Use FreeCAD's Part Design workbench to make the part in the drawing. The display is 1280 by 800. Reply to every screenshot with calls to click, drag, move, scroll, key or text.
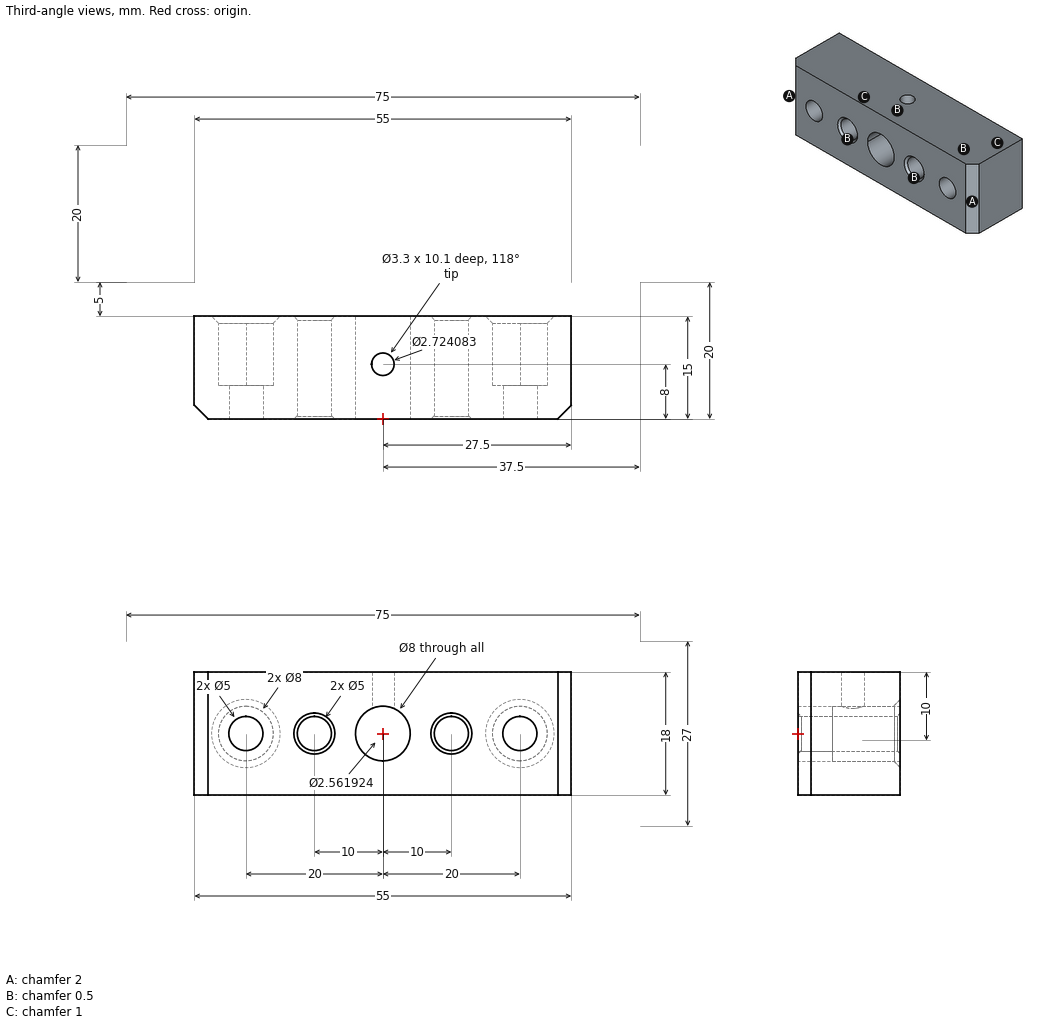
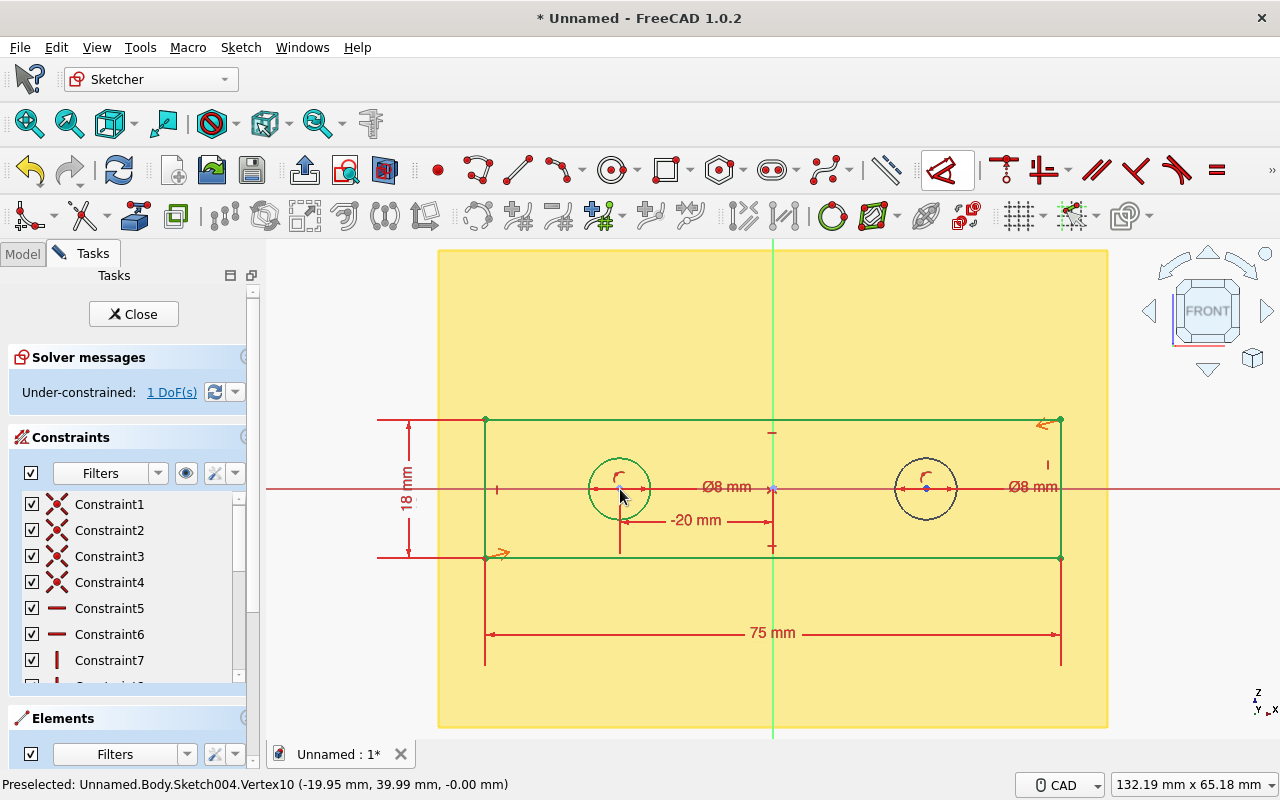
click(926, 489)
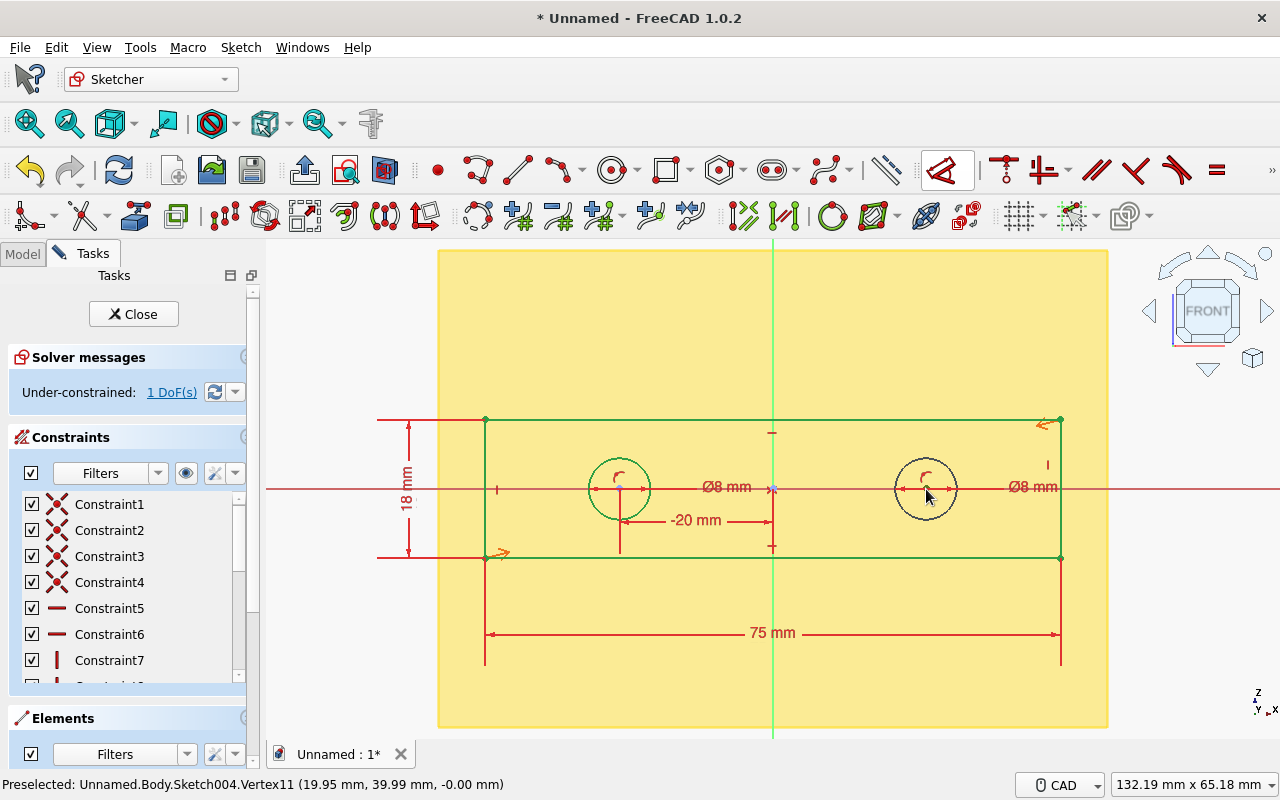
click(968, 170)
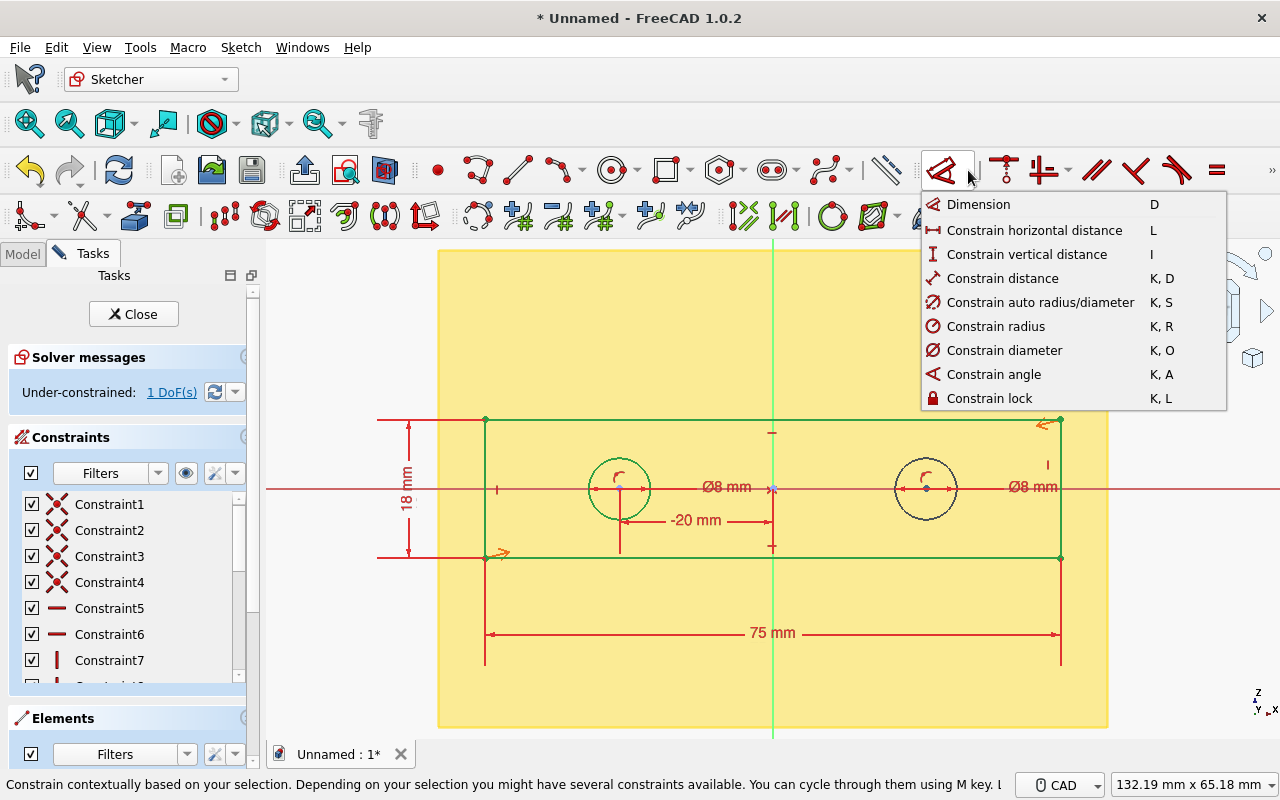
click(1074, 230)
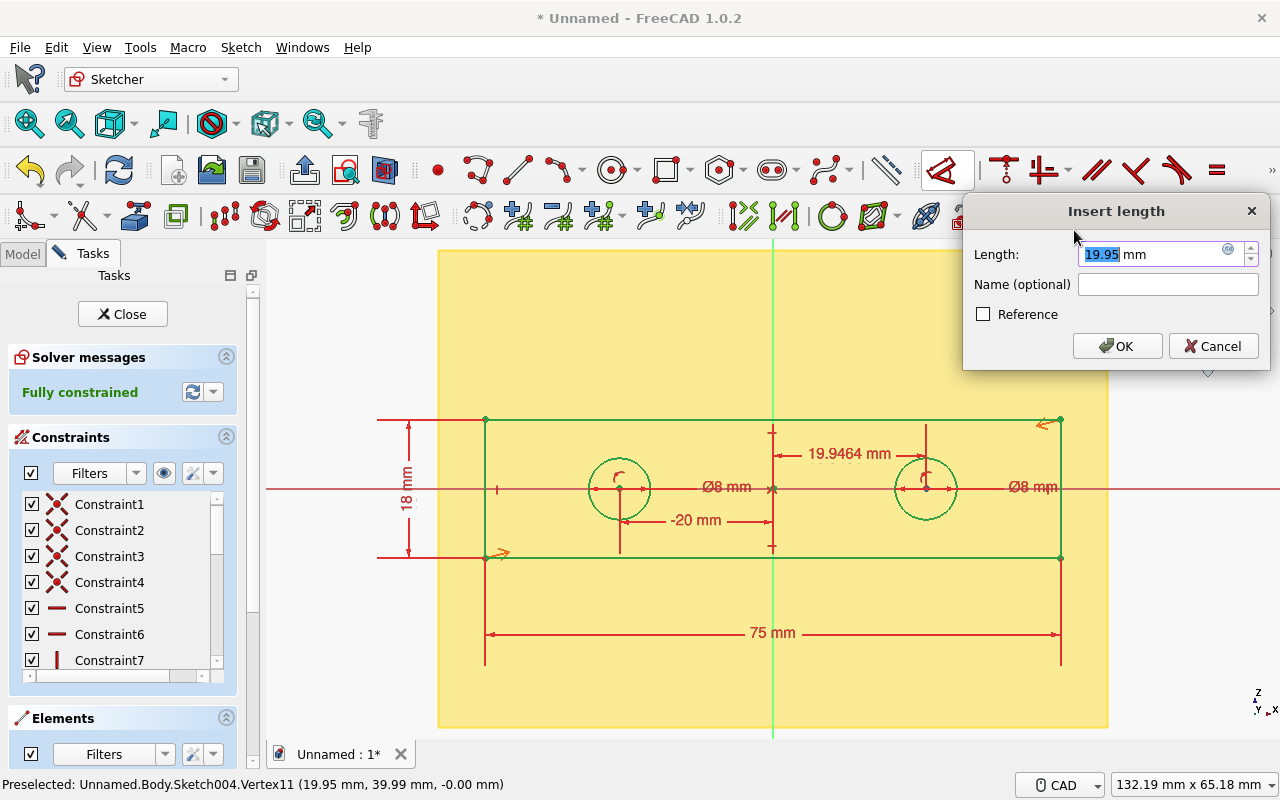
text(20)
key(Return)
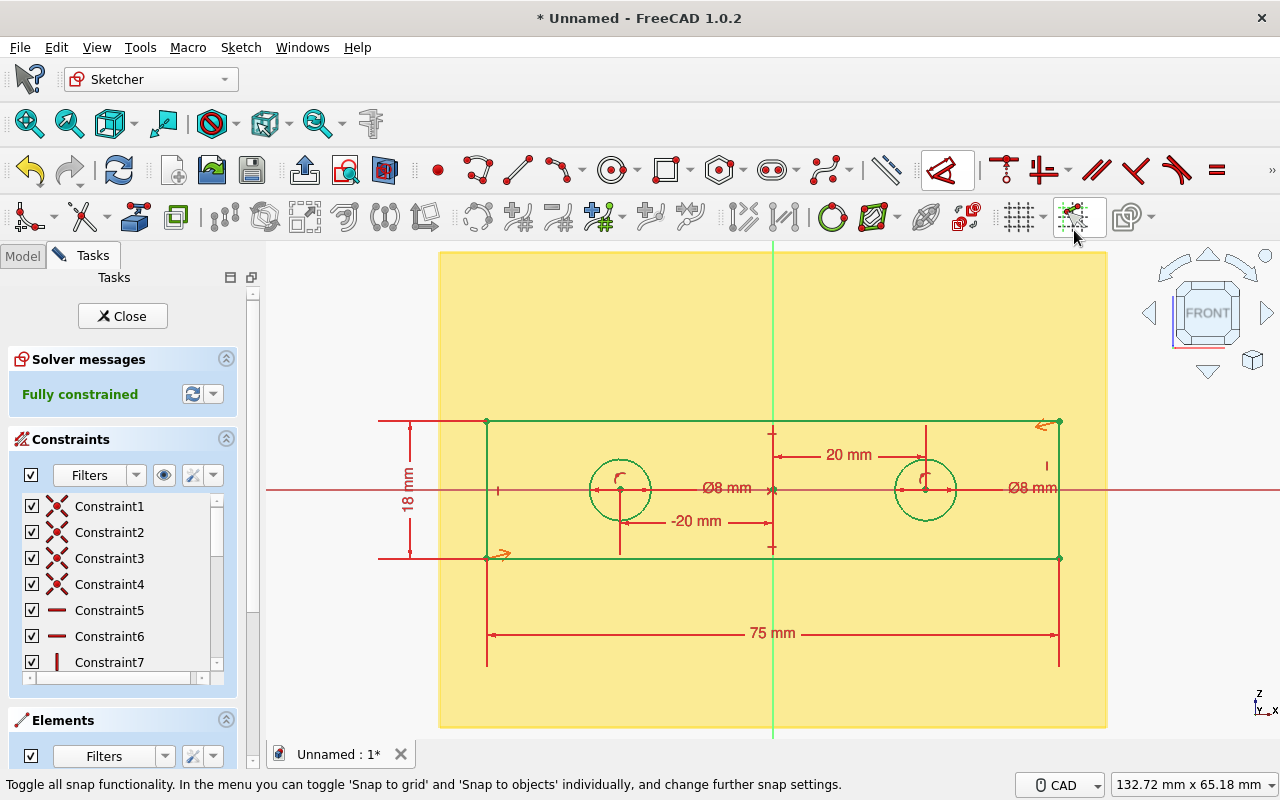
click(123, 316)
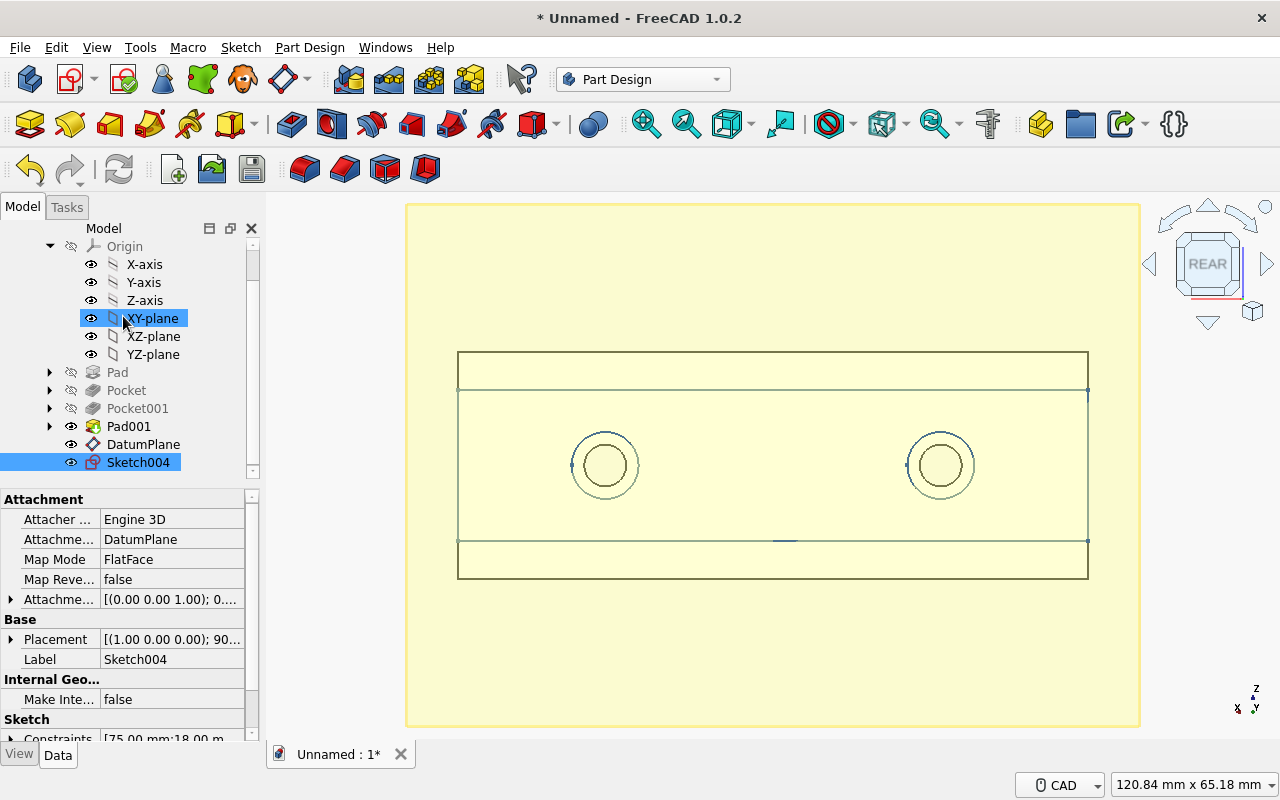
click(30, 124)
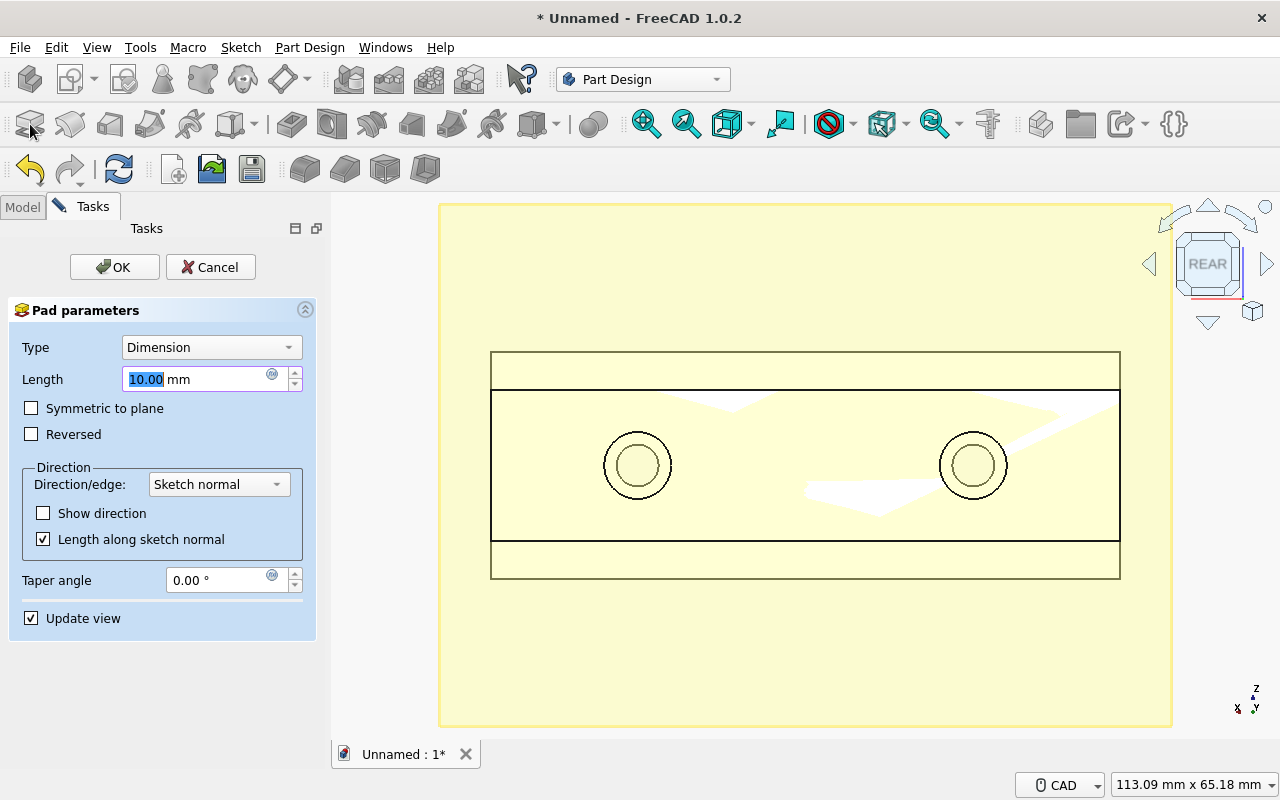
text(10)
key(Tab)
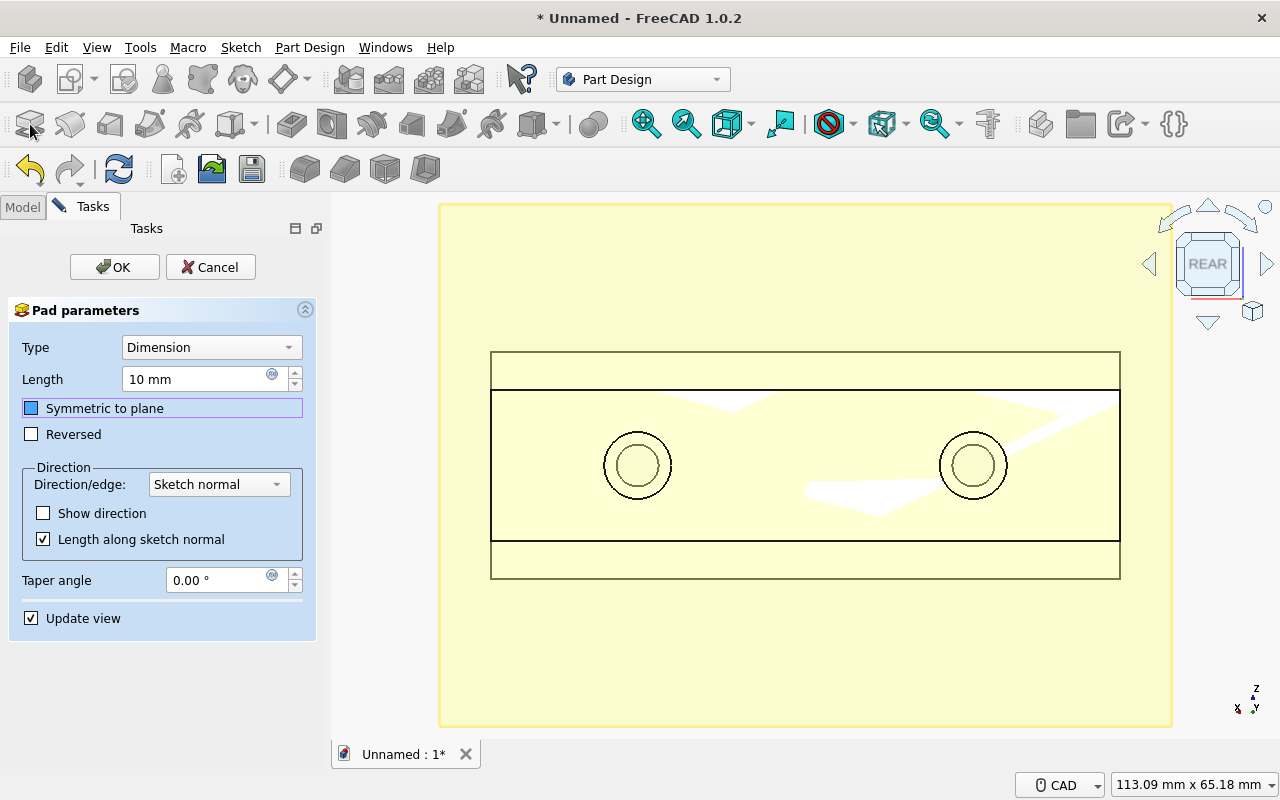
click(115, 267)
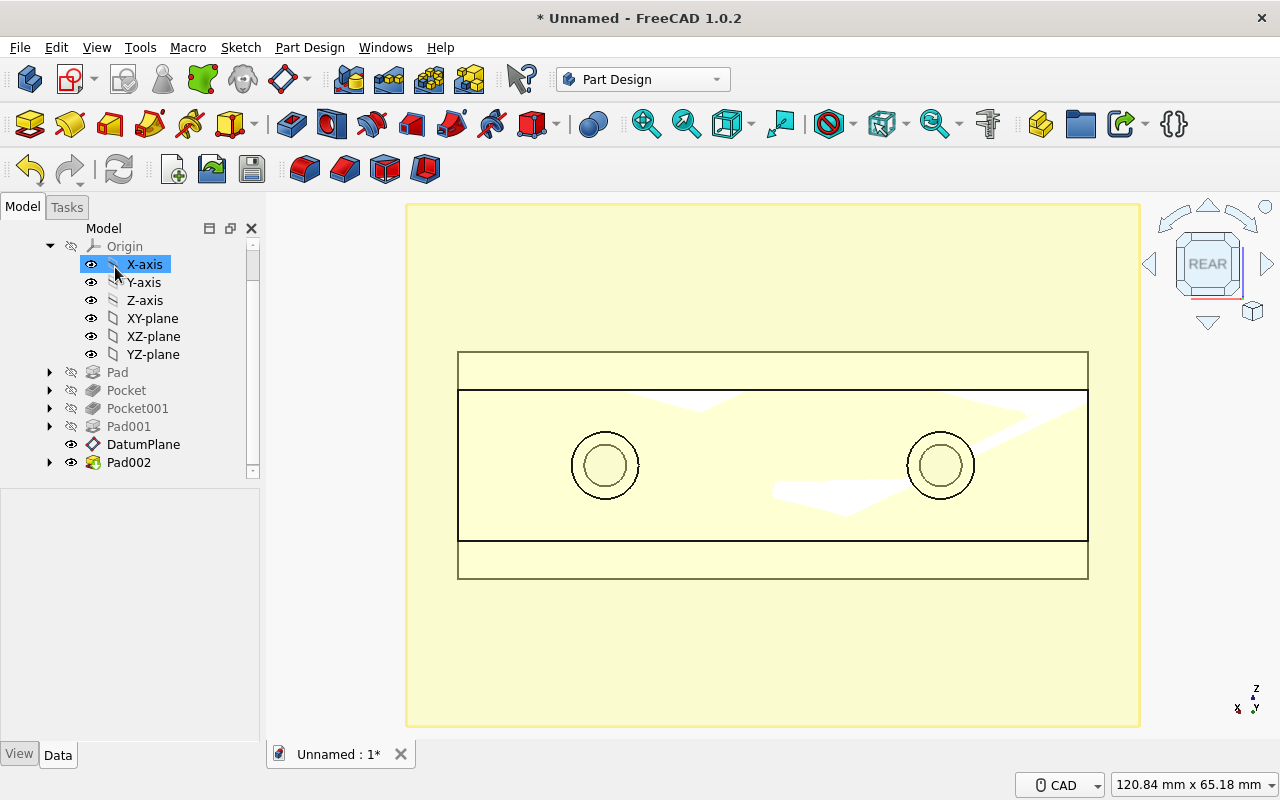
click(116, 444)
key(space)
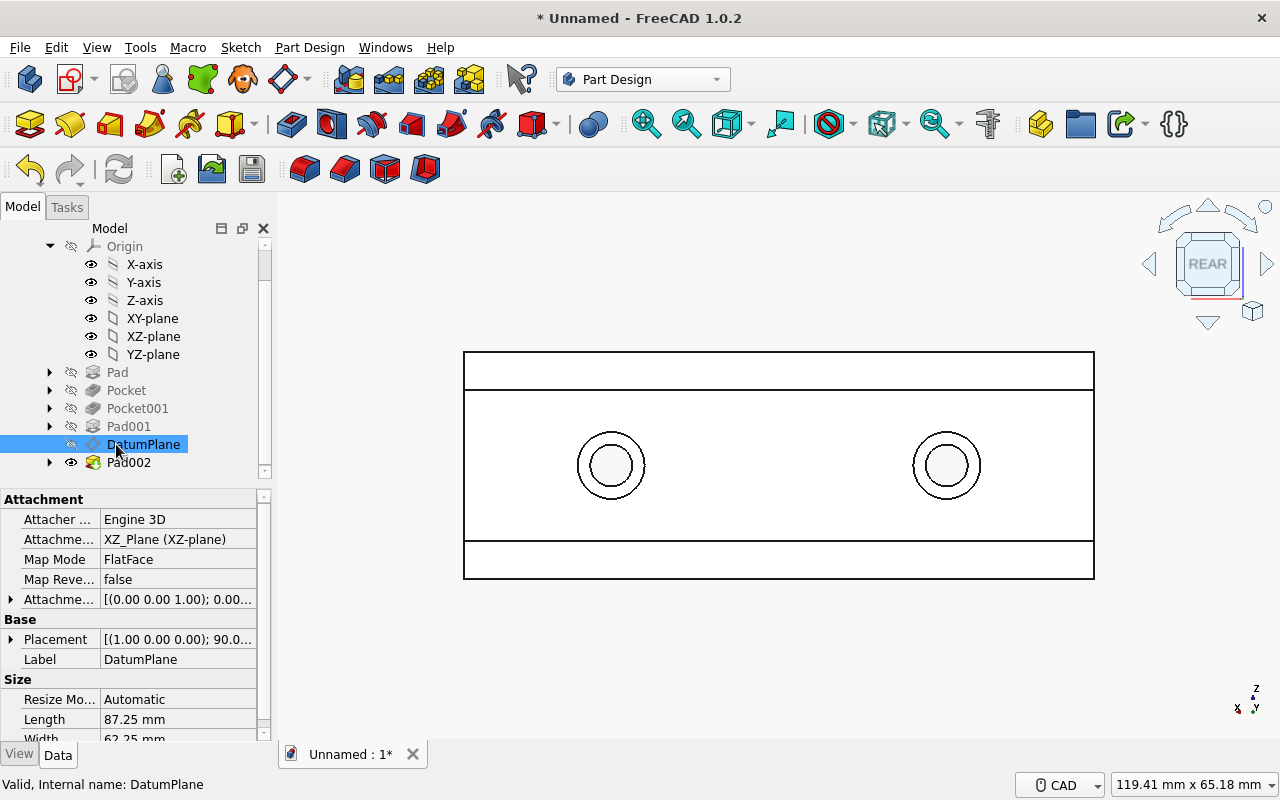
key(0)